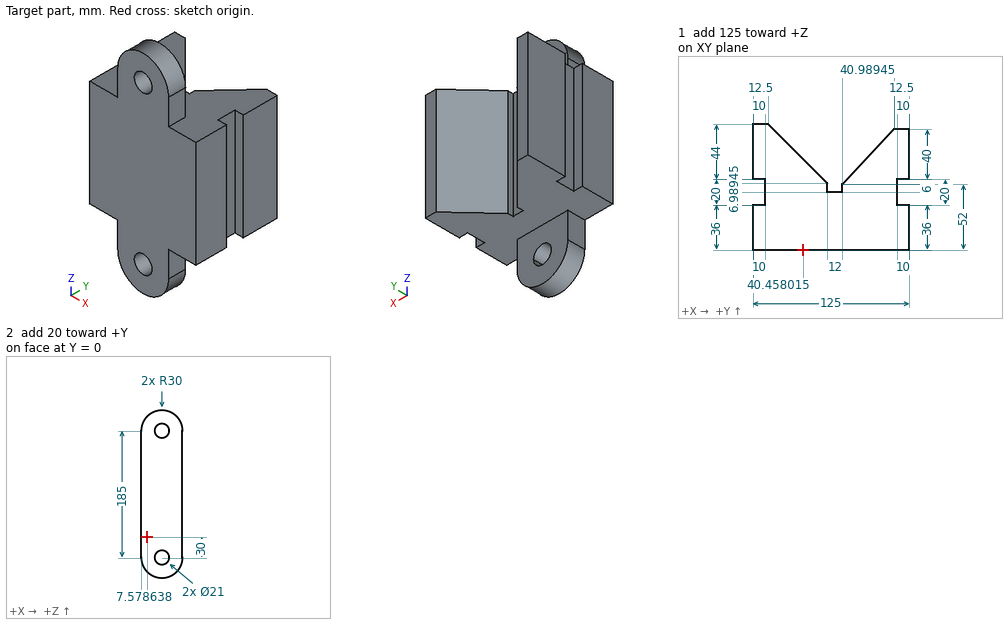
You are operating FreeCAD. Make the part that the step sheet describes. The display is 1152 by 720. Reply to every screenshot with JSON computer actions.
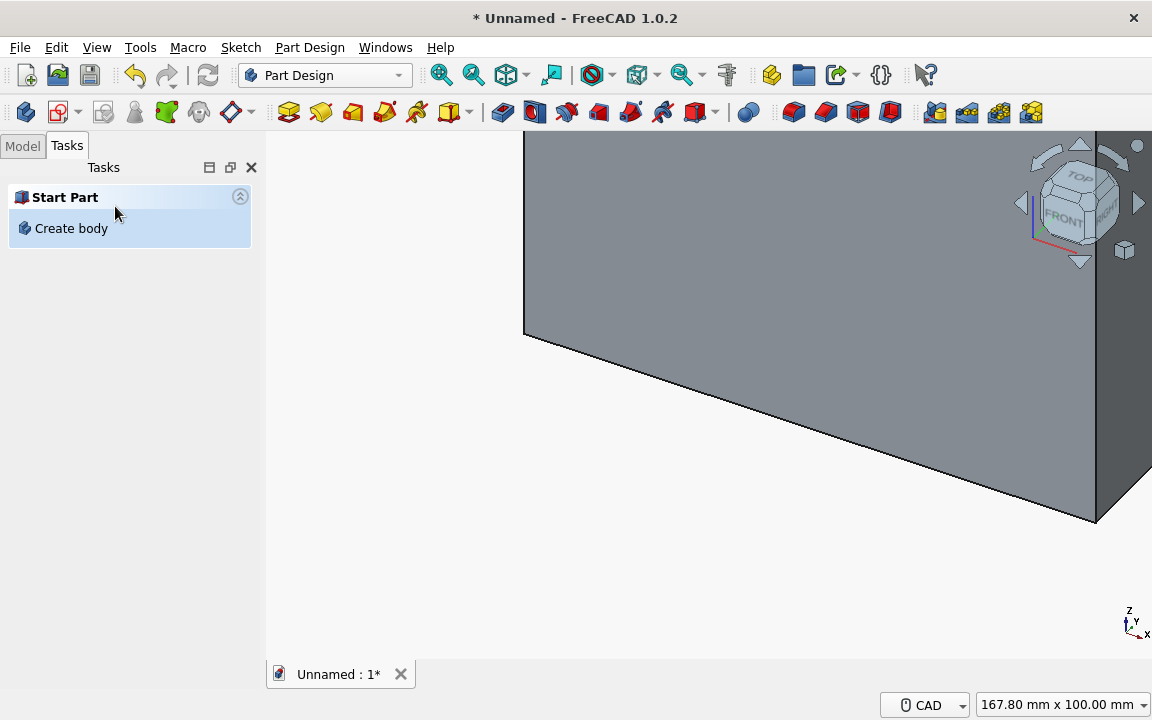
{"action": "key", "text": "v f"}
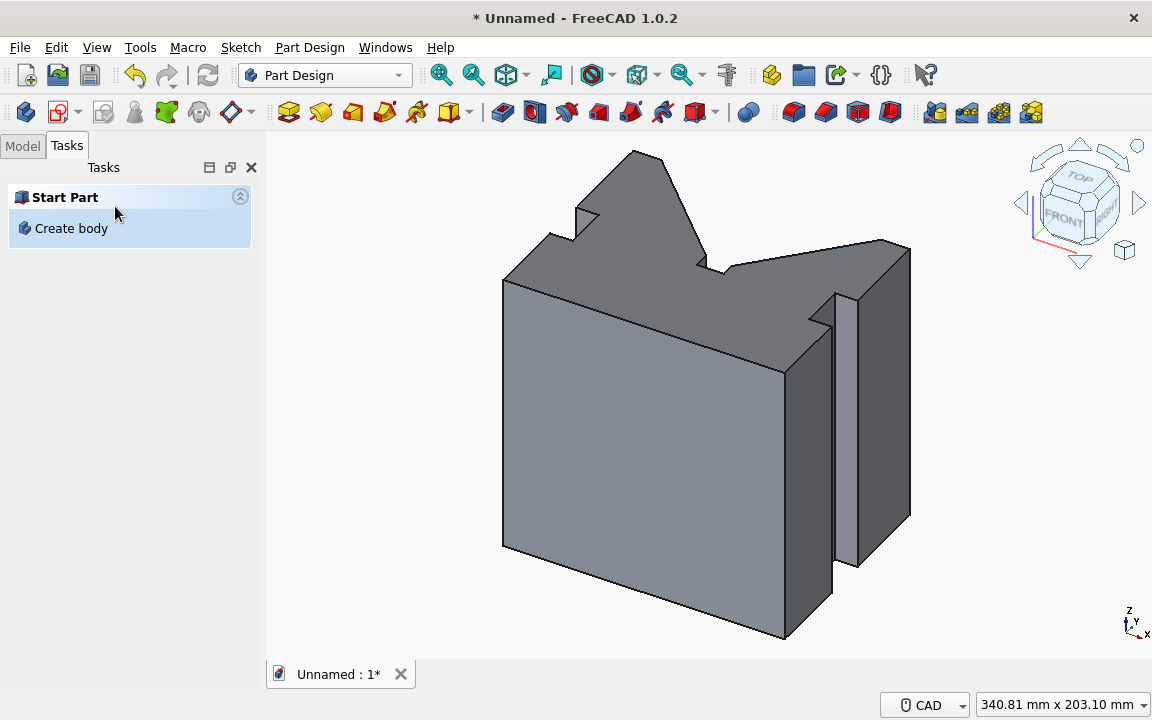
{"action": "left_click", "coordinate": [644, 459]}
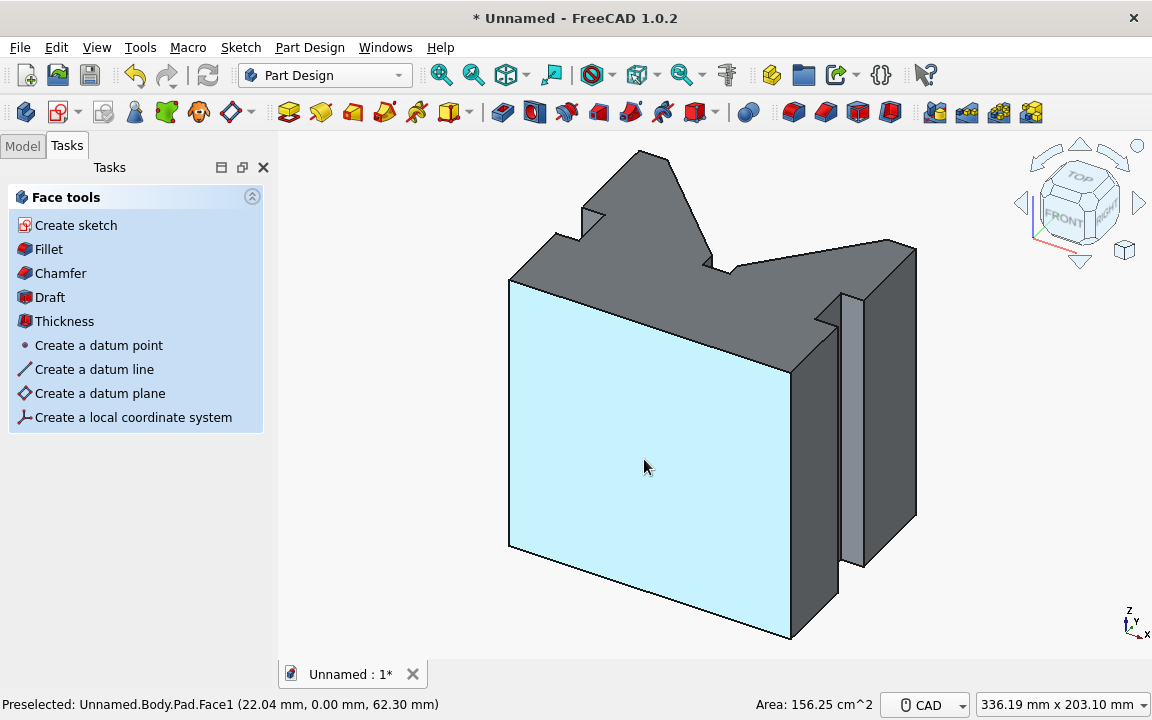
{"action": "left_click", "coordinate": [58, 112]}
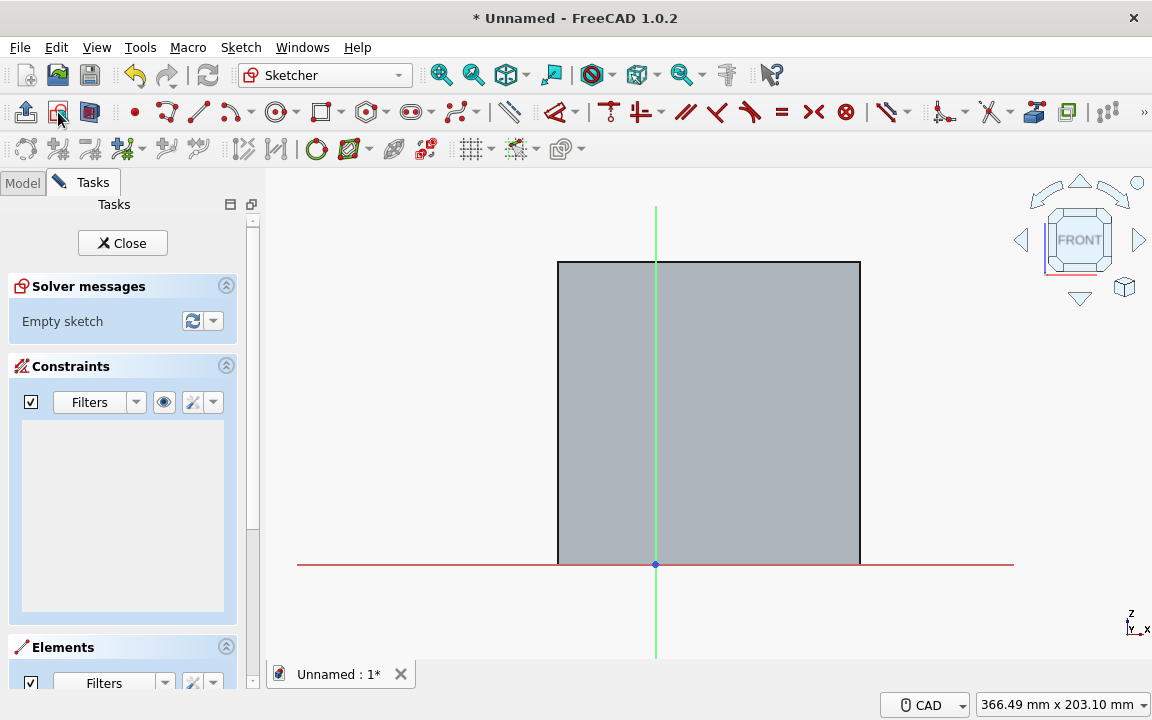
{"action": "scroll", "coordinate": [556, 413], "scroll_direction": "down", "scroll_amount": 3}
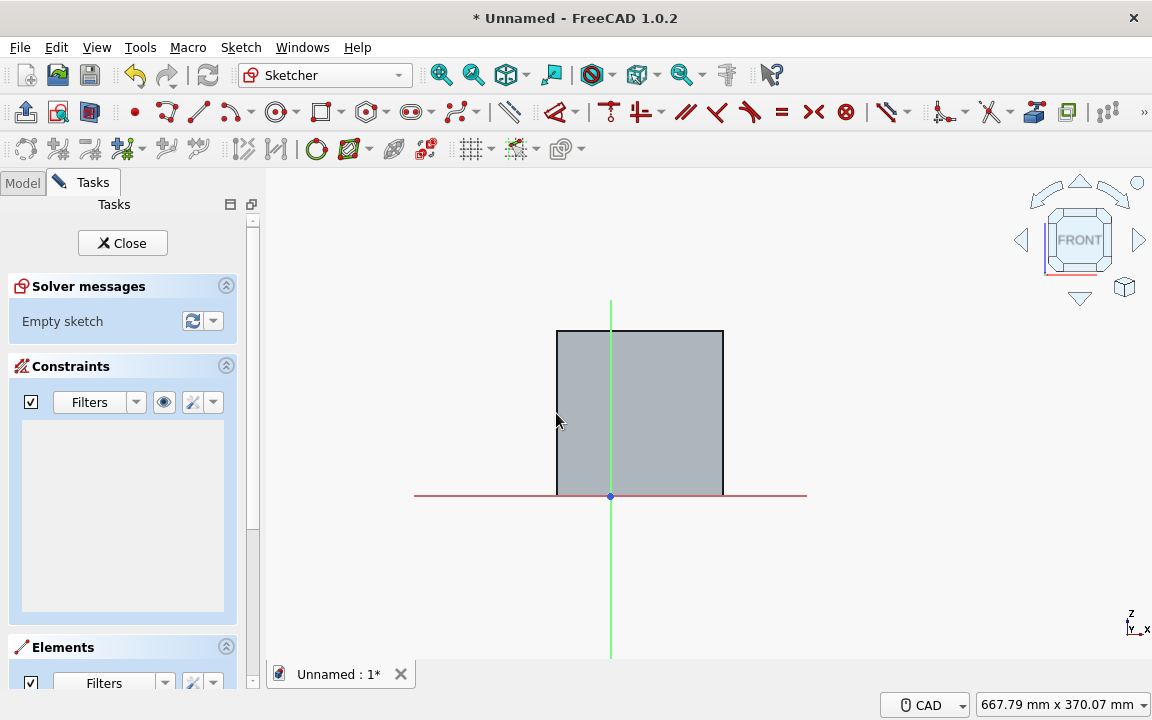
{"action": "key", "text": "g s"}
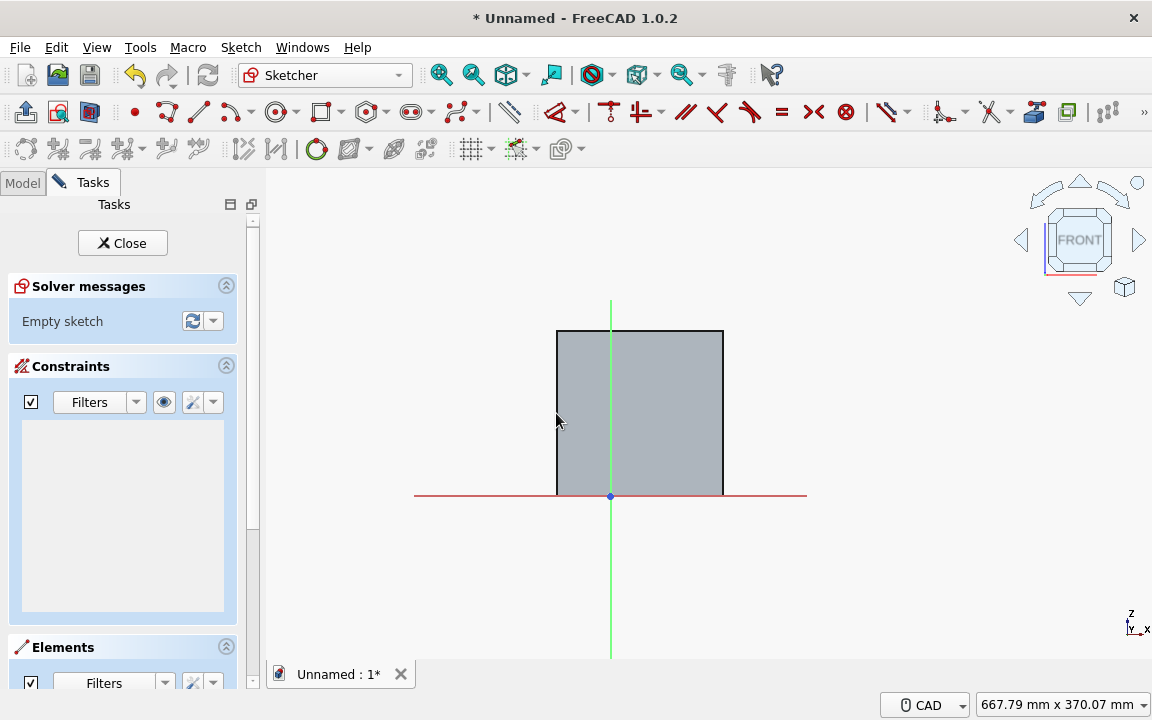
{"action": "left_click", "coordinate": [641, 536]}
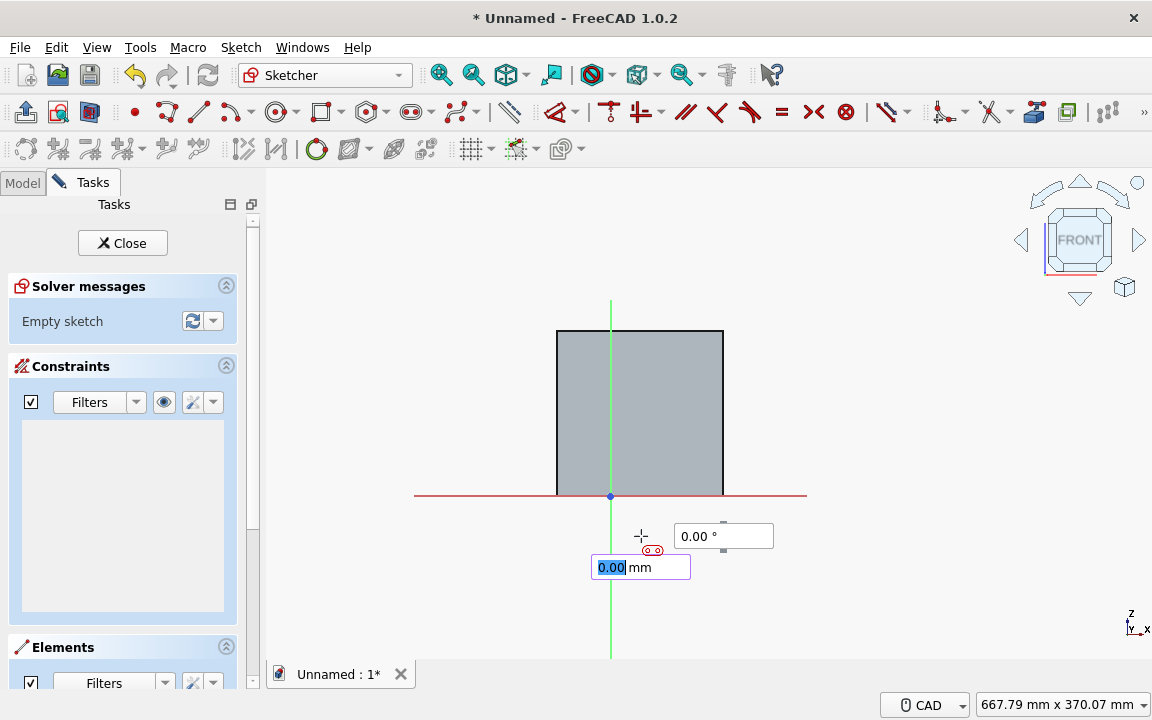
{"action": "left_click", "coordinate": [641, 291]}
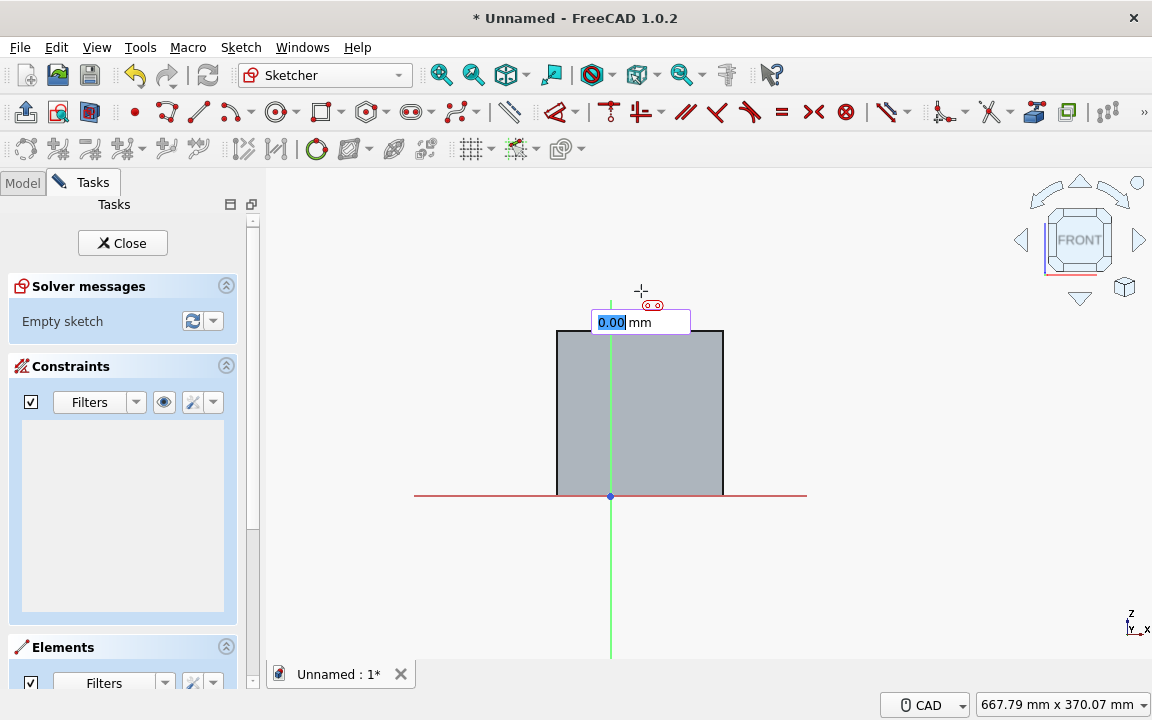
{"action": "left_click", "coordinate": [680, 414]}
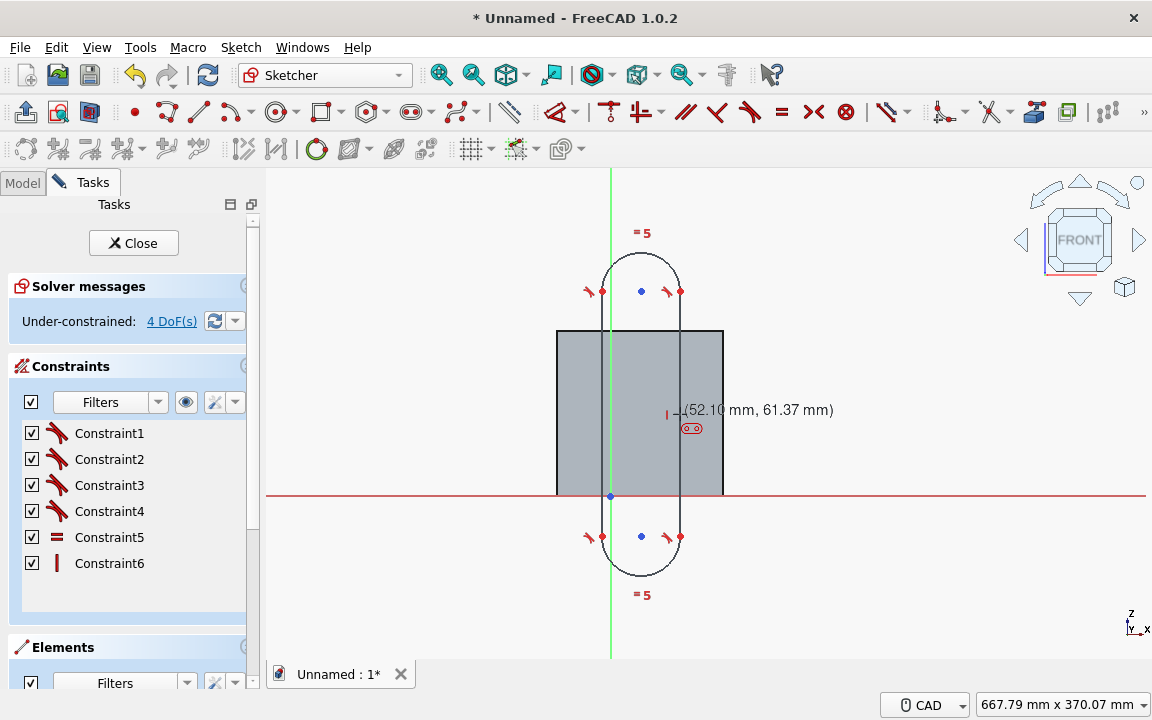
{"action": "key", "text": "g c"}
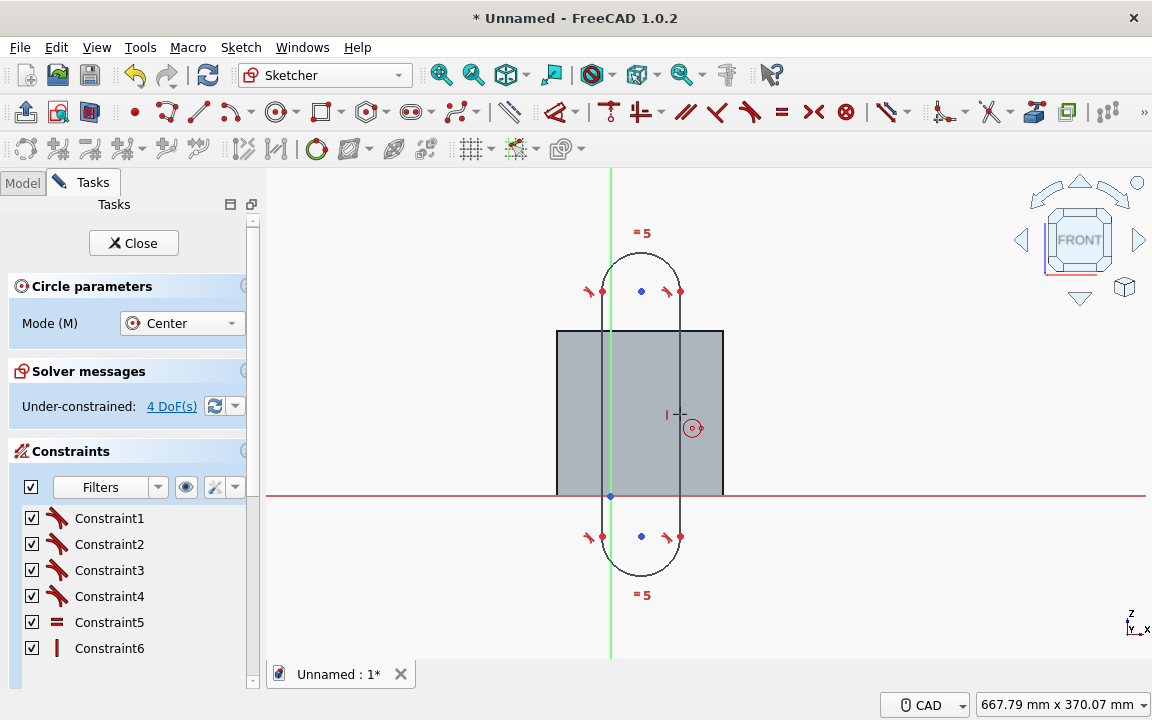
{"action": "scroll", "coordinate": [641, 536], "scroll_direction": "up", "scroll_amount": 3}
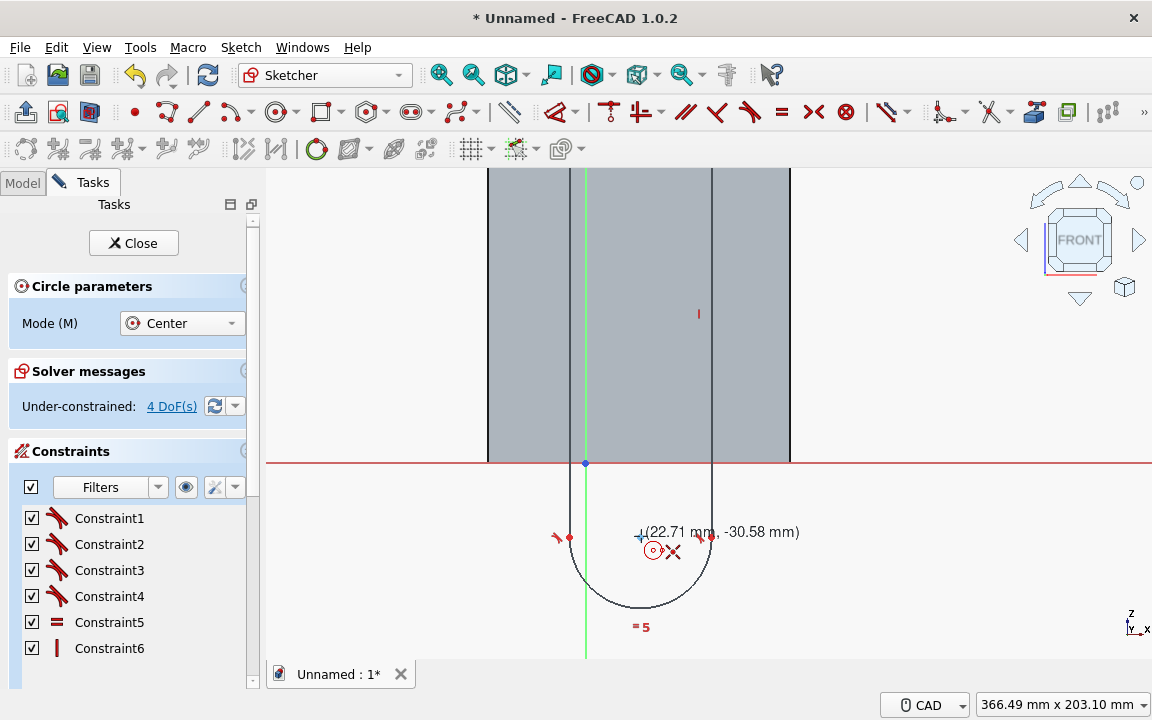
{"action": "left_click", "coordinate": [641, 537]}
{"action": "mouse_move", "coordinate": [658, 518]}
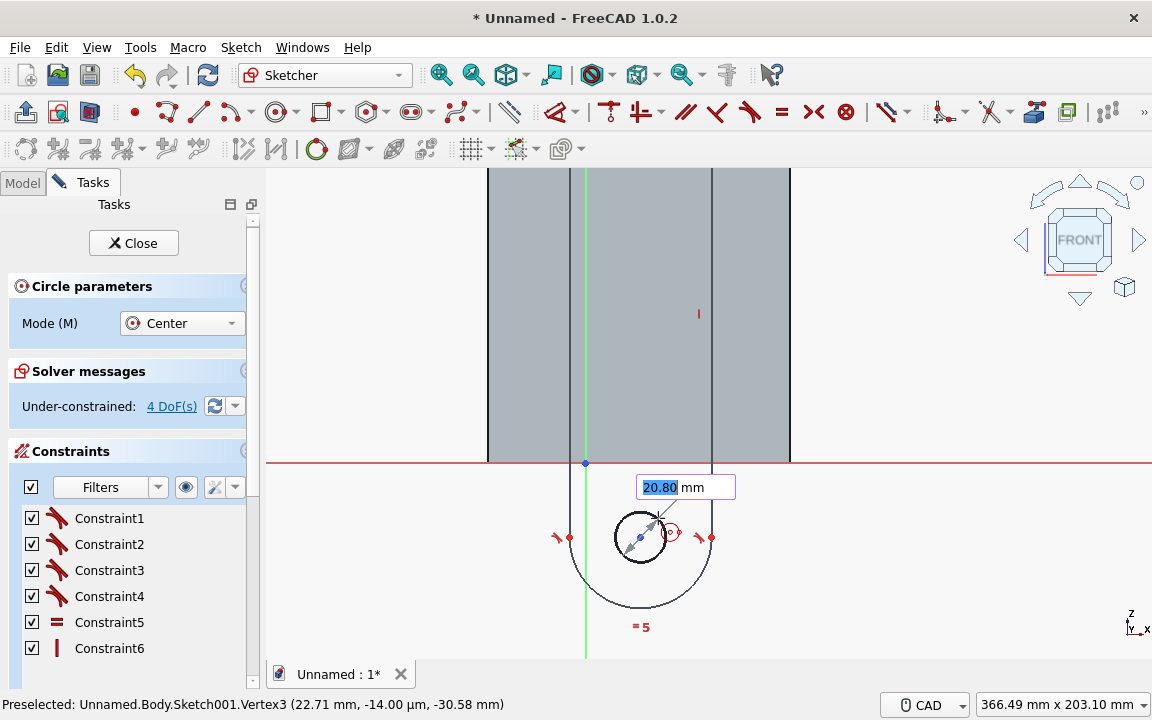
{"action": "type", "text": "21"}
{"action": "key", "text": "Return"}